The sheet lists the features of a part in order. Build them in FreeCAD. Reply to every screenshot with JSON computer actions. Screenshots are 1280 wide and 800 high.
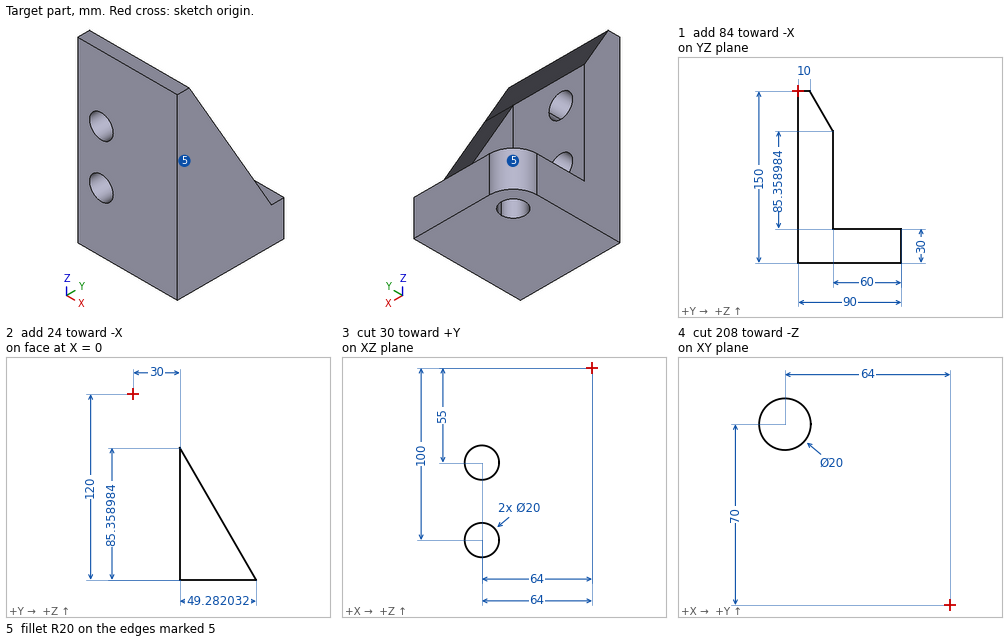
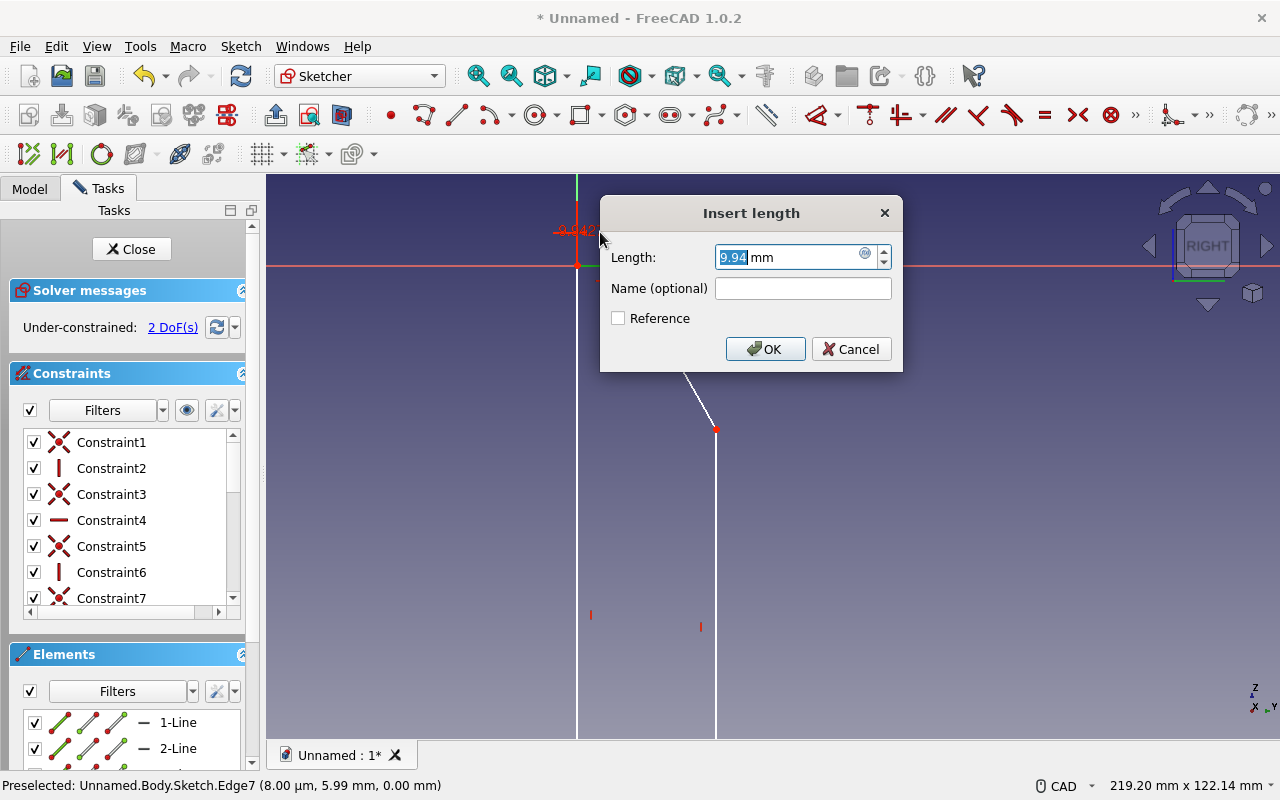
{"action": "type", "text": "10"}
{"action": "key", "text": "Return"}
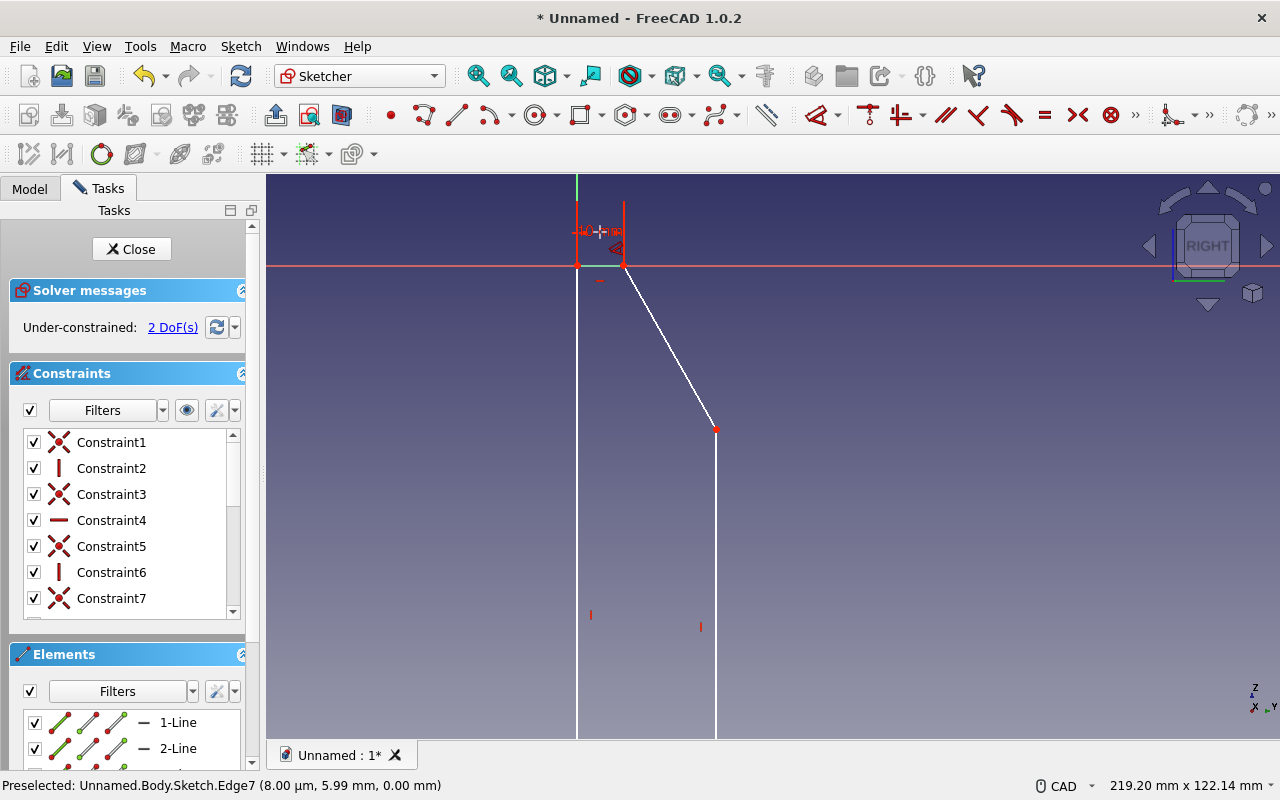
{"action": "left_click", "coordinate": [577, 475]}
{"action": "left_click", "coordinate": [543, 488]}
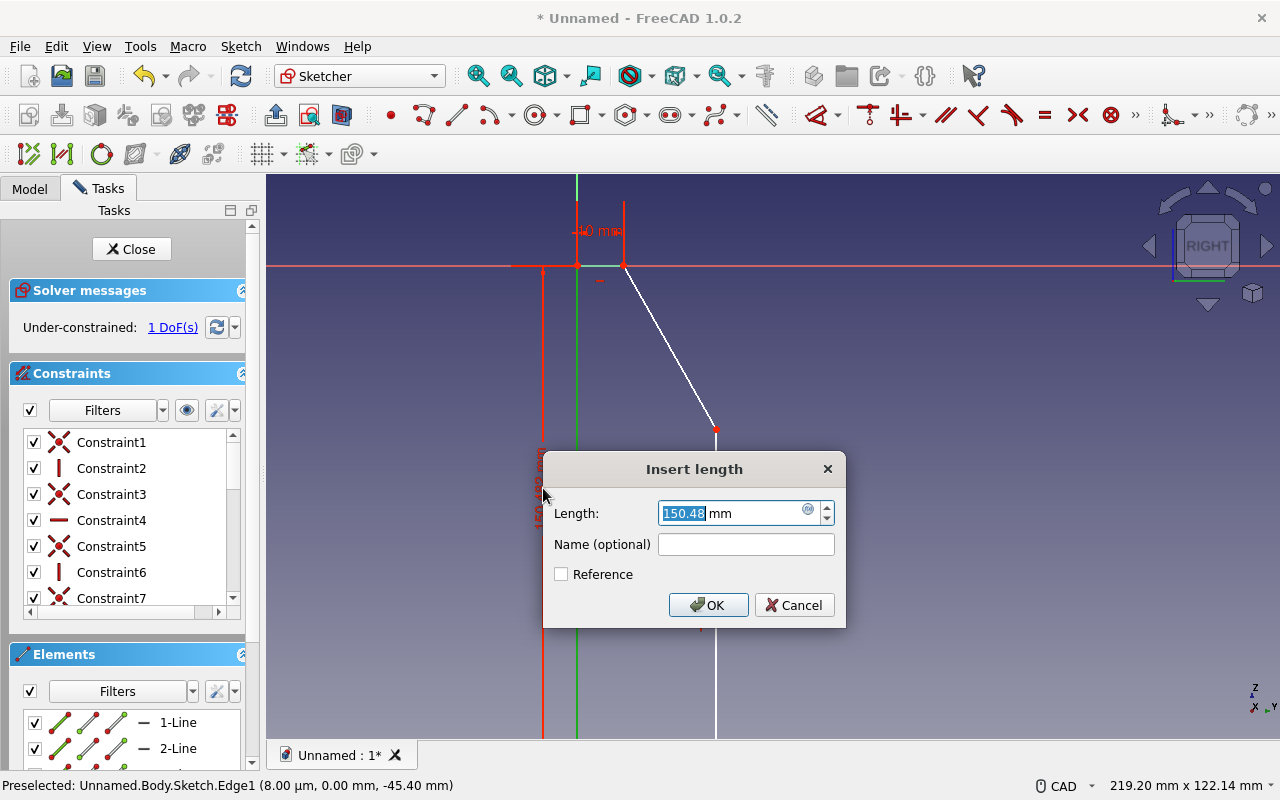
{"action": "type", "text": "150"}
{"action": "key", "text": "Return"}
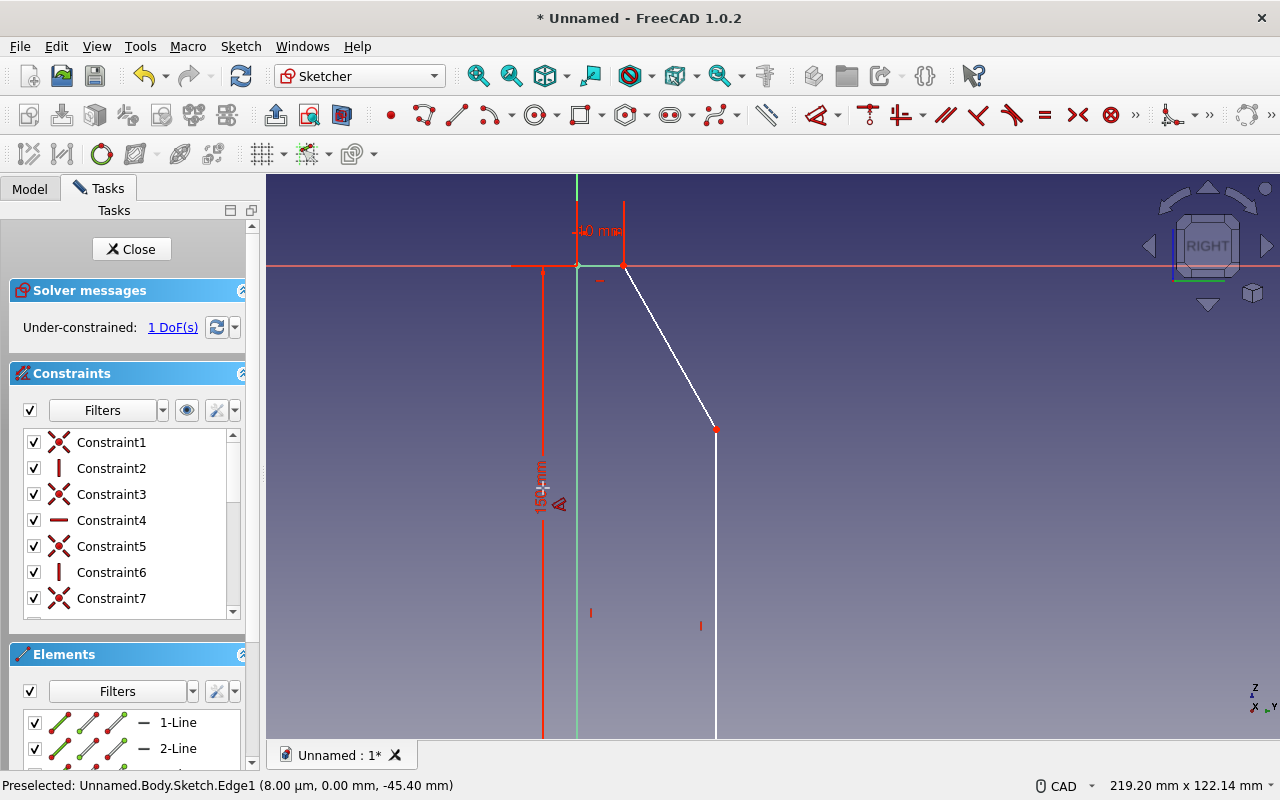
{"action": "left_click", "coordinate": [716, 703]}
{"action": "left_click", "coordinate": [682, 570]}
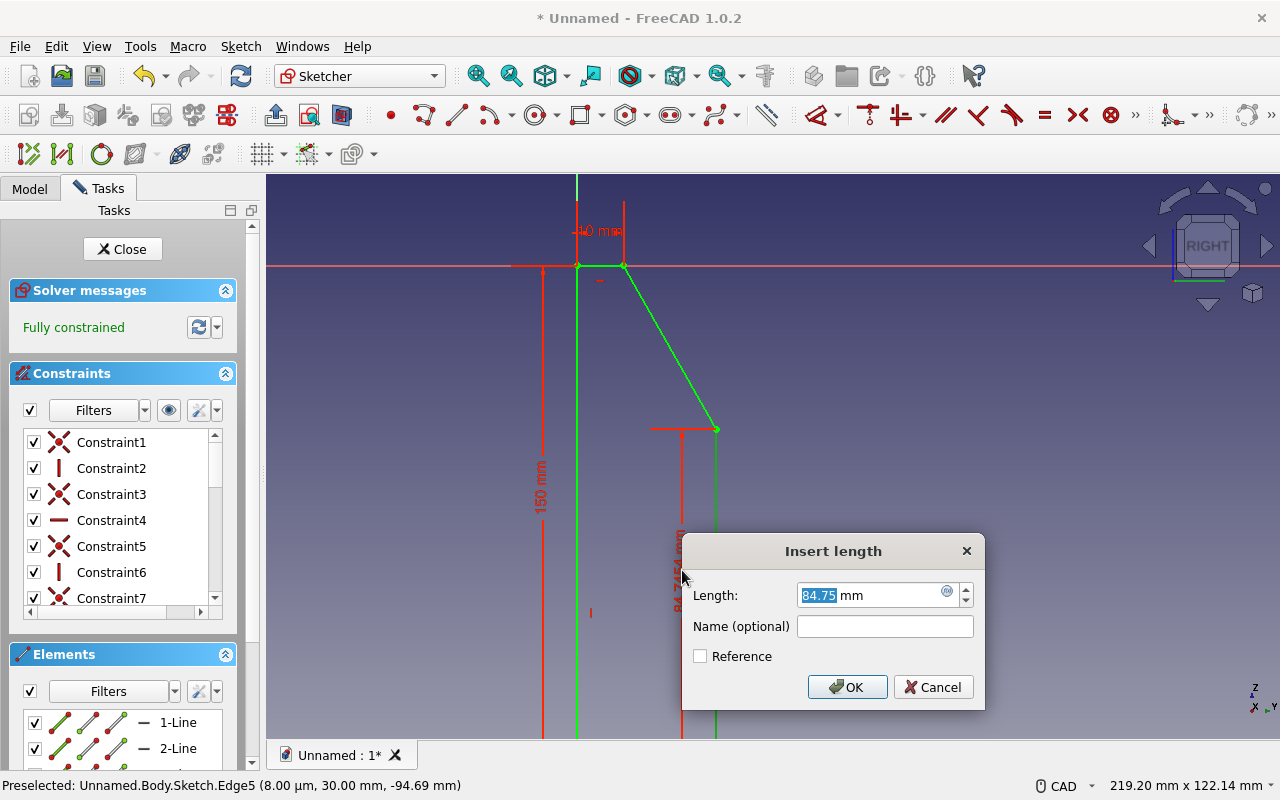
{"action": "type", "text": "85.358984"}
{"action": "key", "text": "Return"}
{"action": "key", "text": "Escape"}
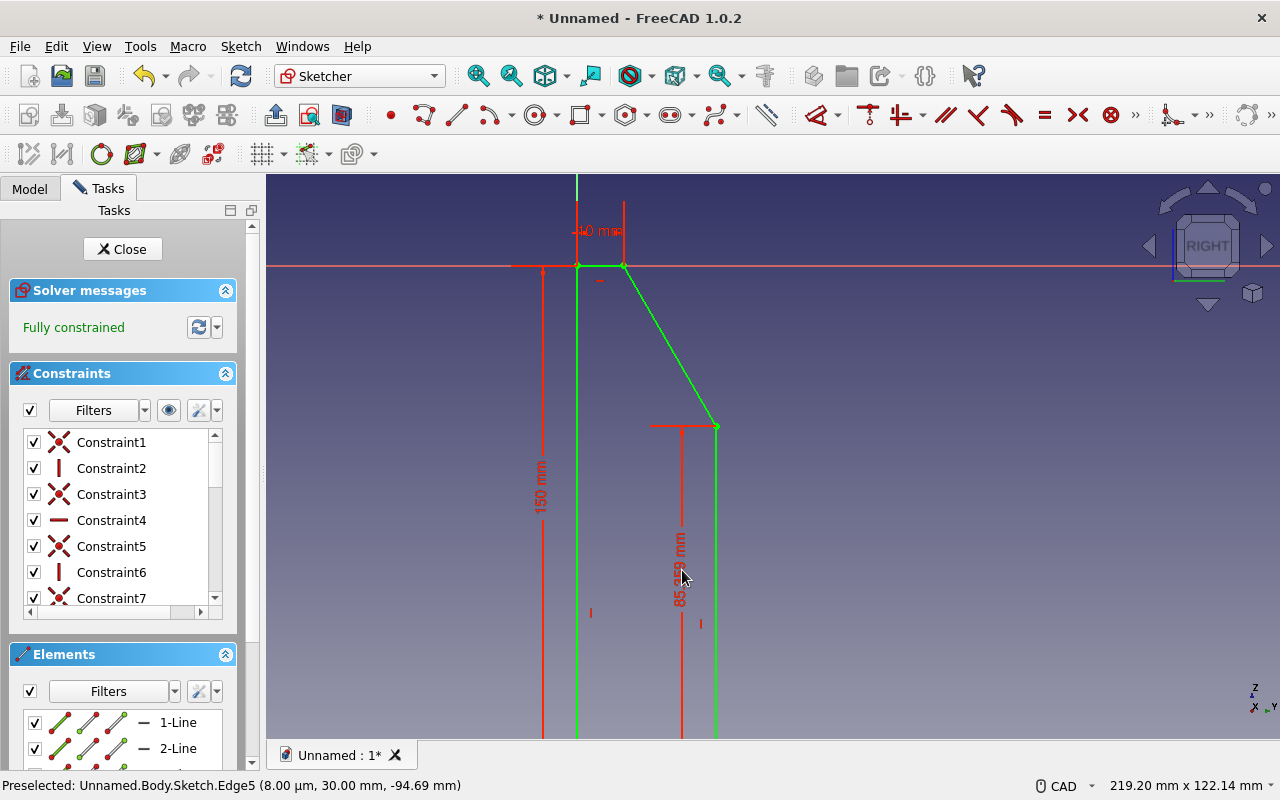
{"action": "left_click", "coordinate": [123, 249]}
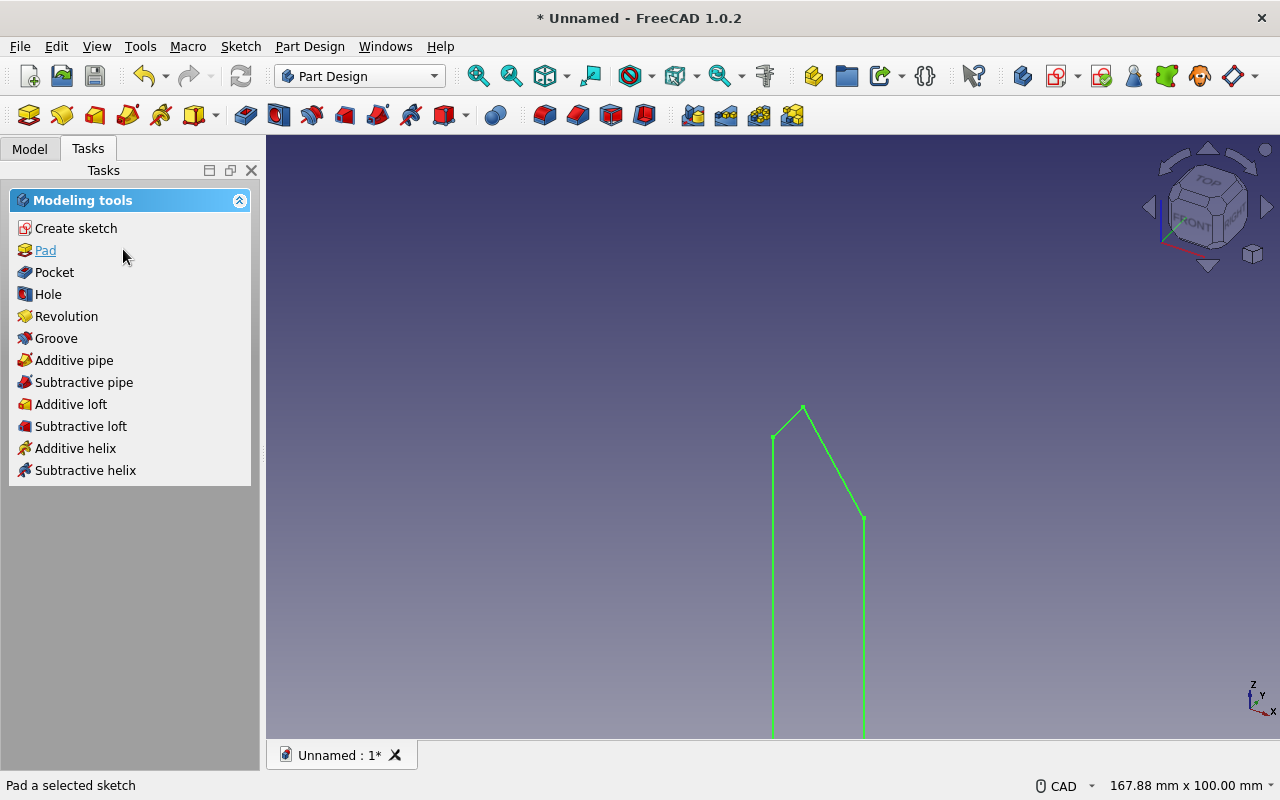
{"action": "left_click", "coordinate": [29, 116]}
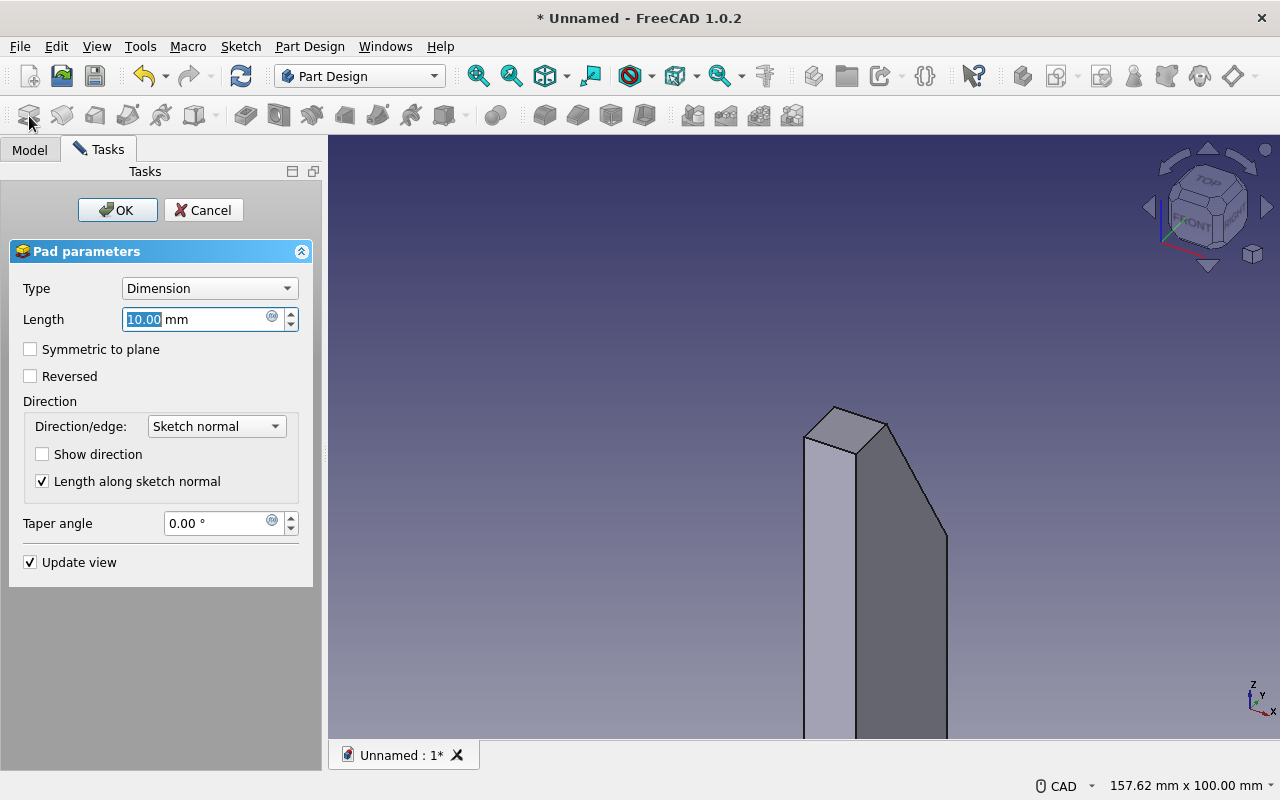
{"action": "type", "text": "84"}
{"action": "key", "text": "Tab"}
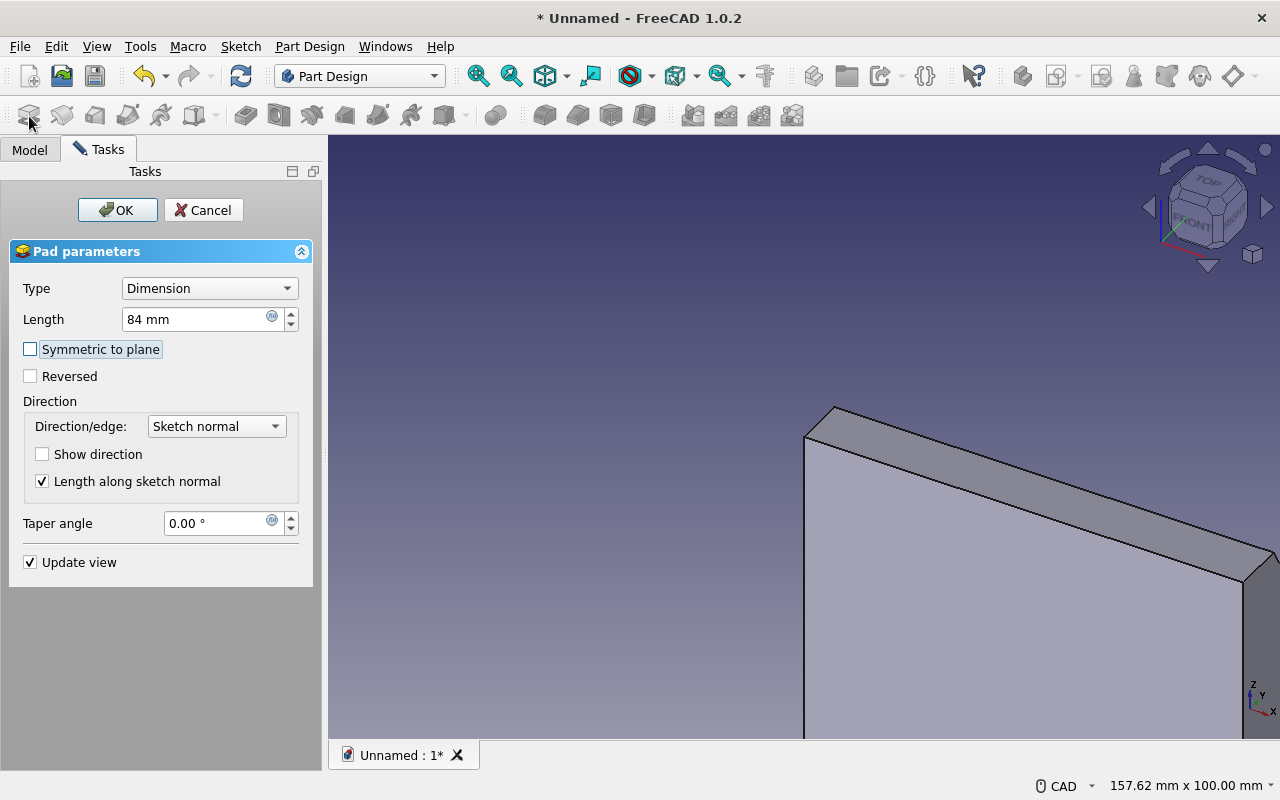
{"action": "left_click", "coordinate": [31, 376]}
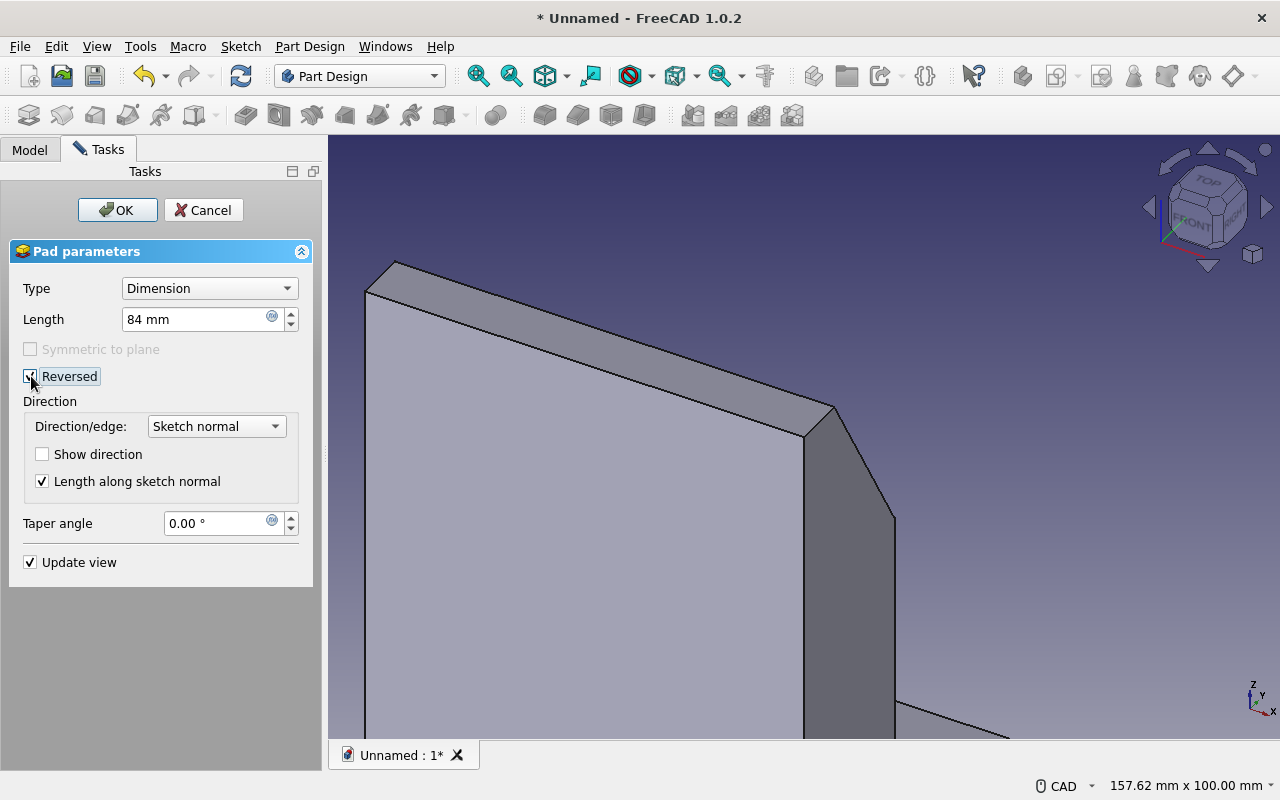
{"action": "left_click", "coordinate": [118, 210]}